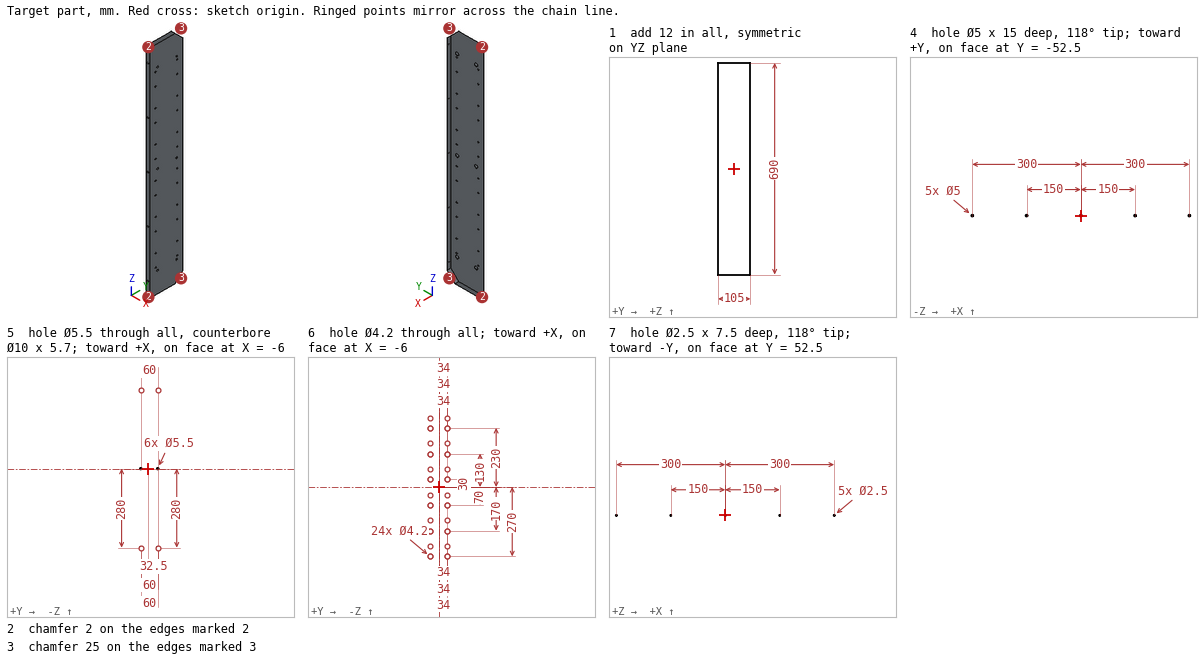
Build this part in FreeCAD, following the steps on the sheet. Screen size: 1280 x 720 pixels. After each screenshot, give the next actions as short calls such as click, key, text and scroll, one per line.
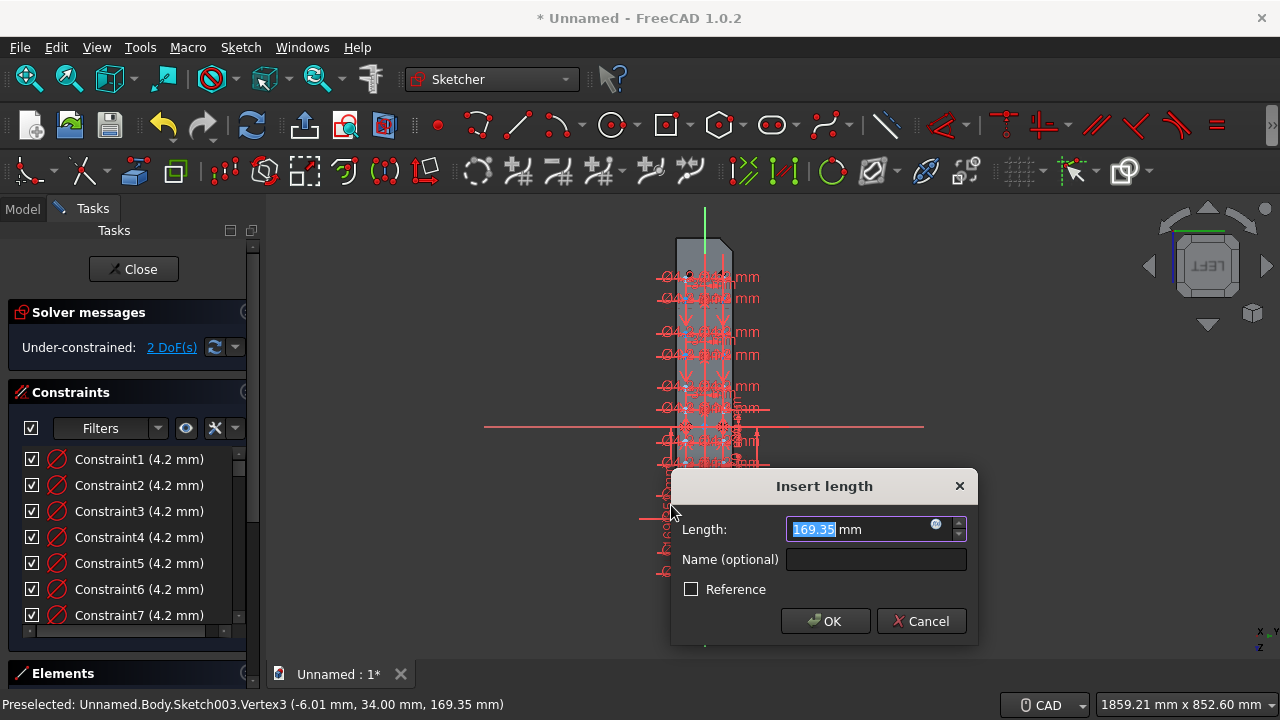
text(170)
key(Return)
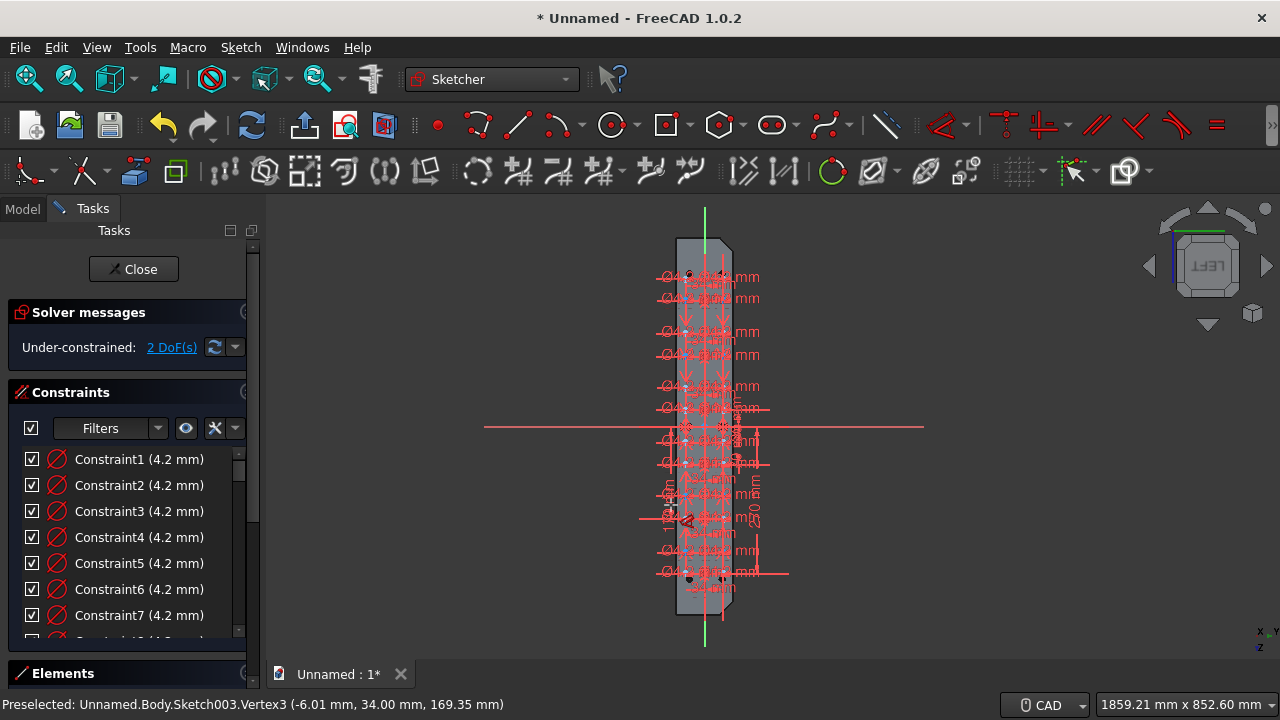
click(723, 357)
click(757, 367)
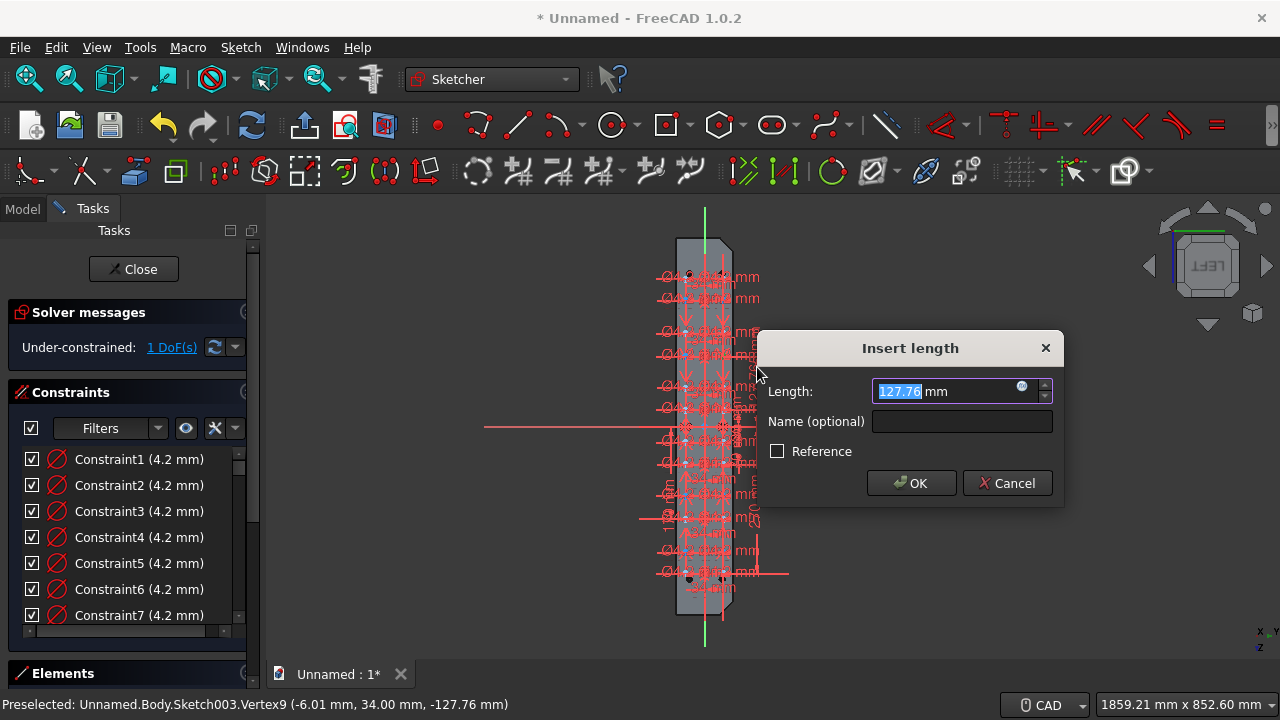
text(130)
key(Return)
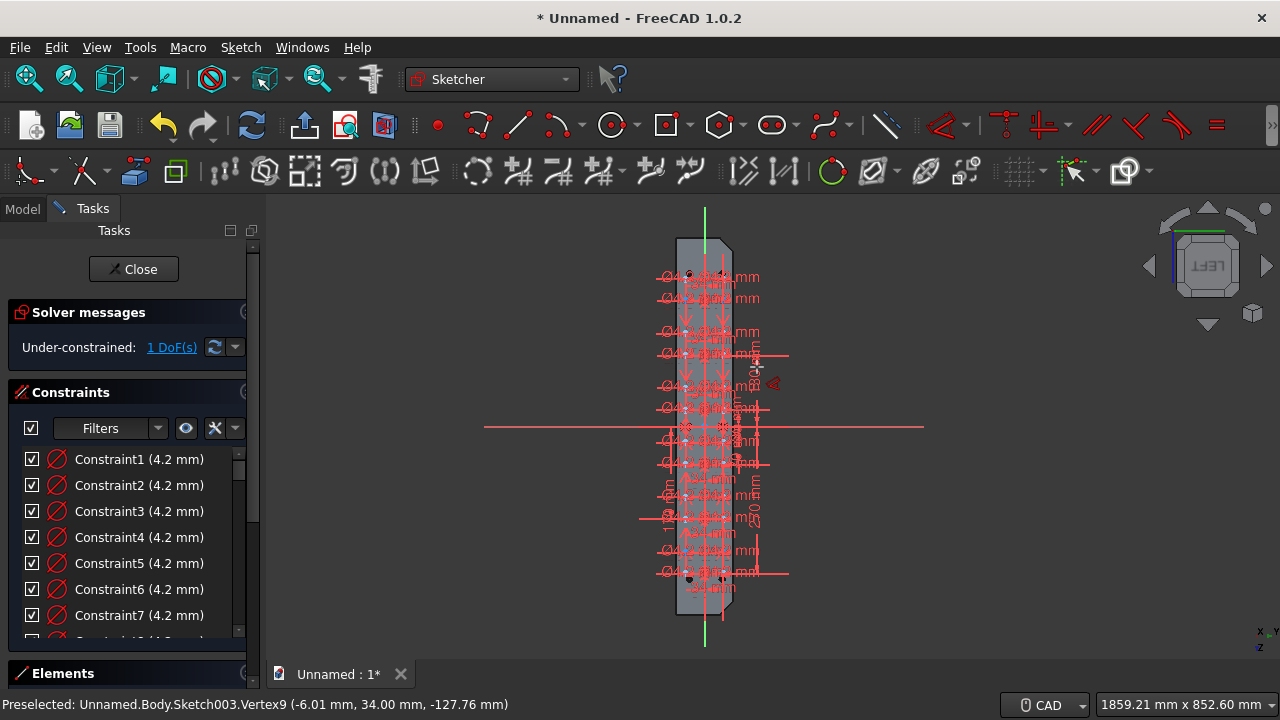
click(723, 301)
click(757, 319)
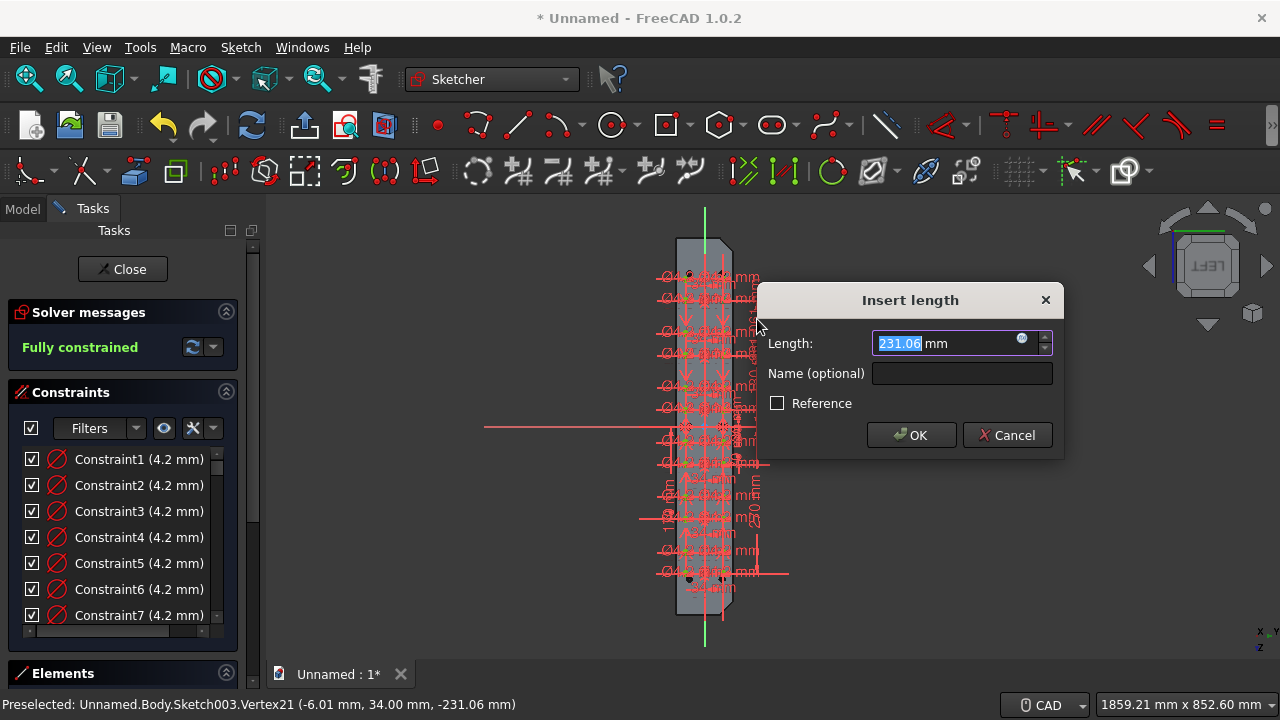
text(230)
key(Return)
key(Escape)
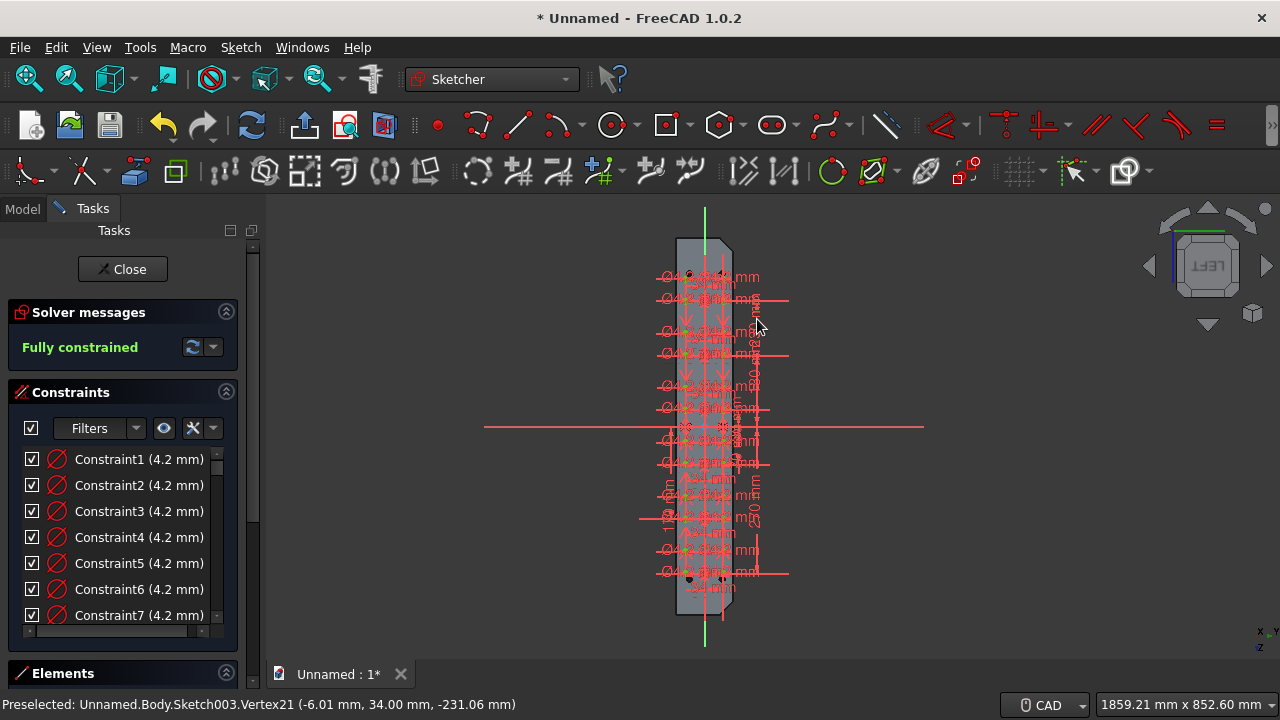
click(123, 269)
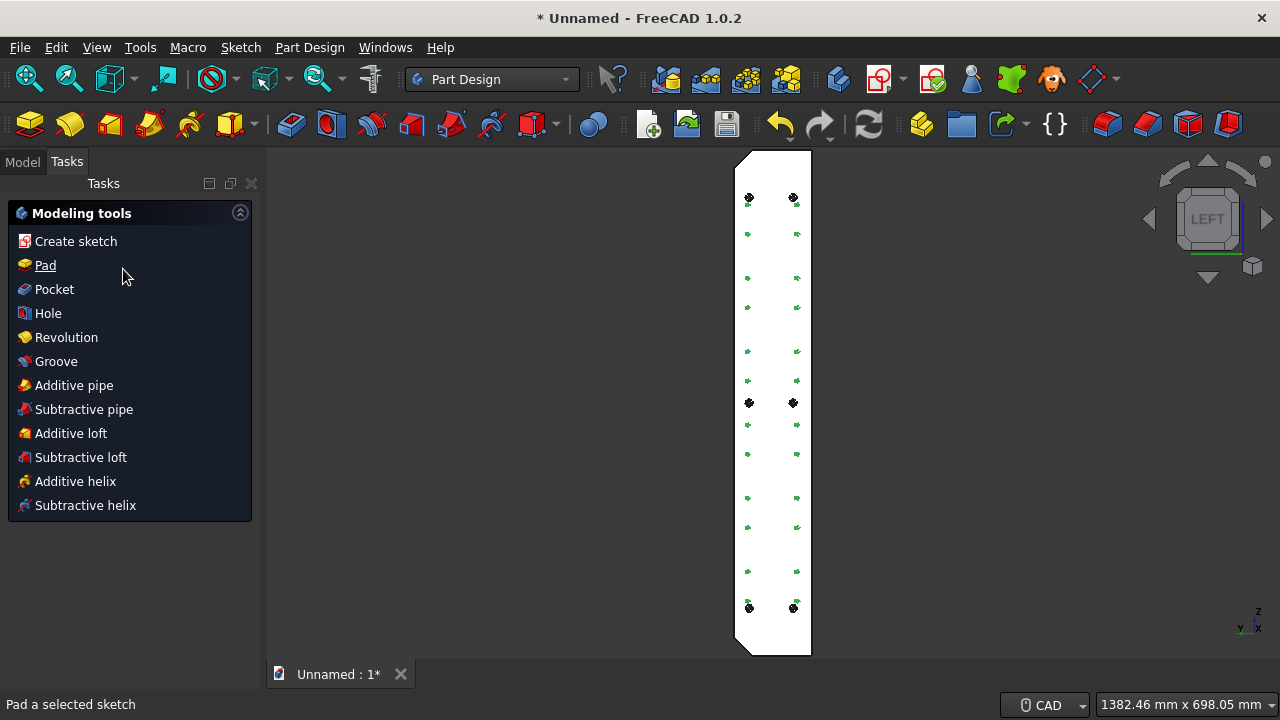
click(332, 124)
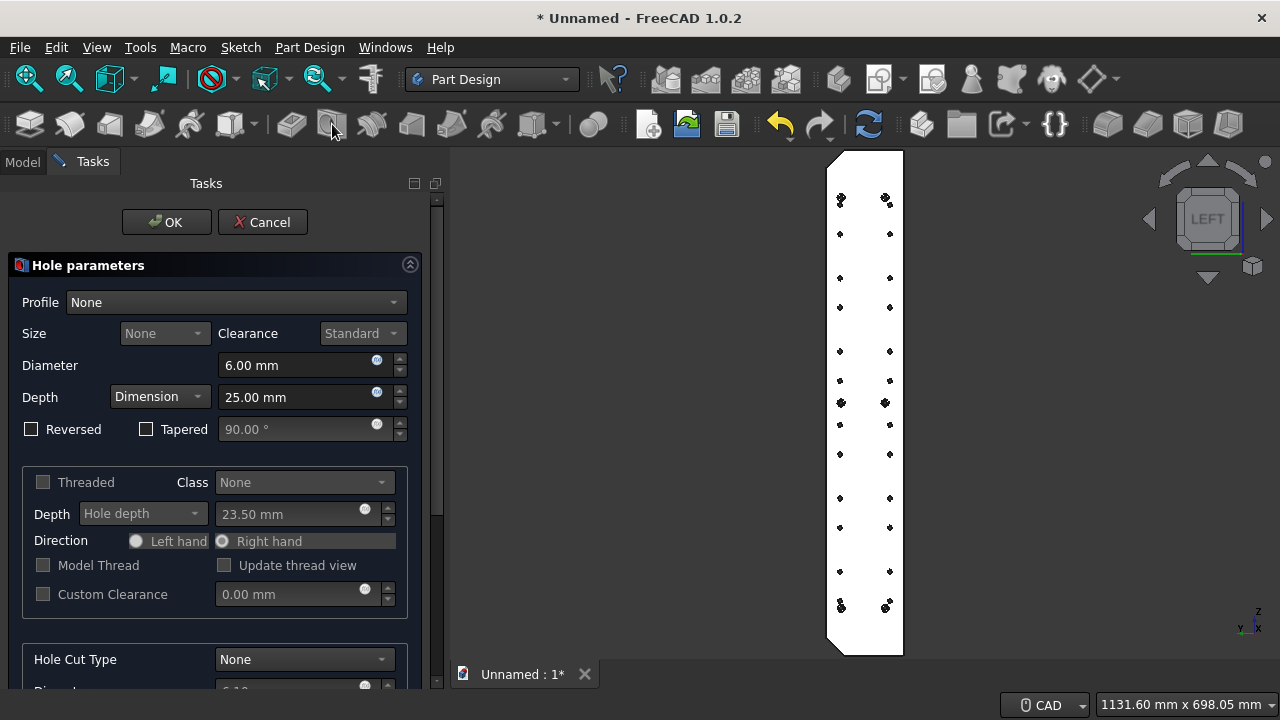
triple_click(305, 365)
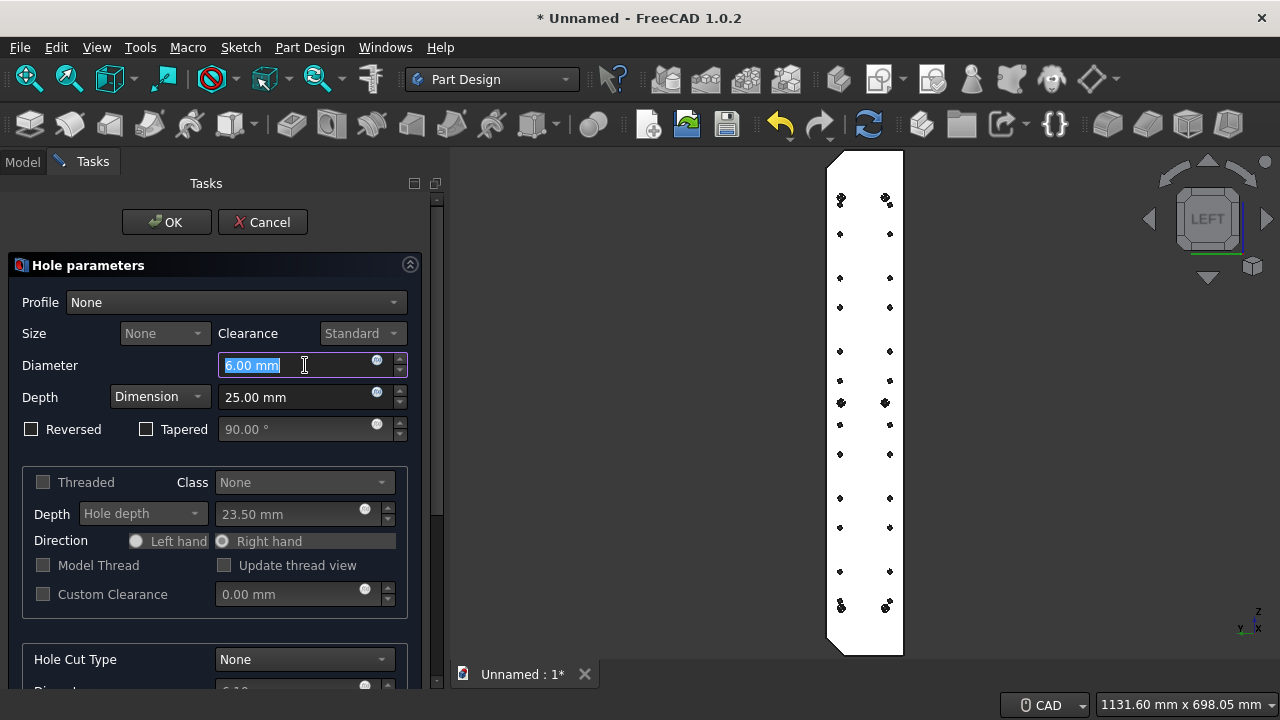
text(4.2)
key(Tab)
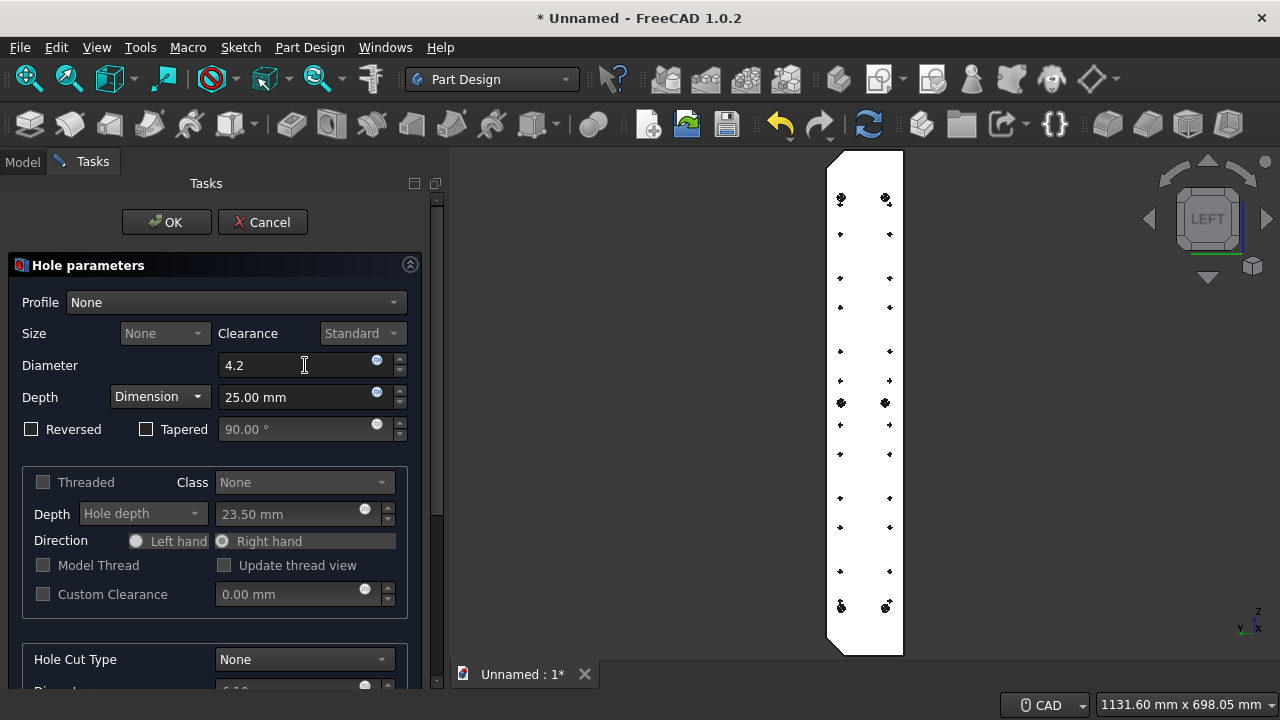
click(161, 396)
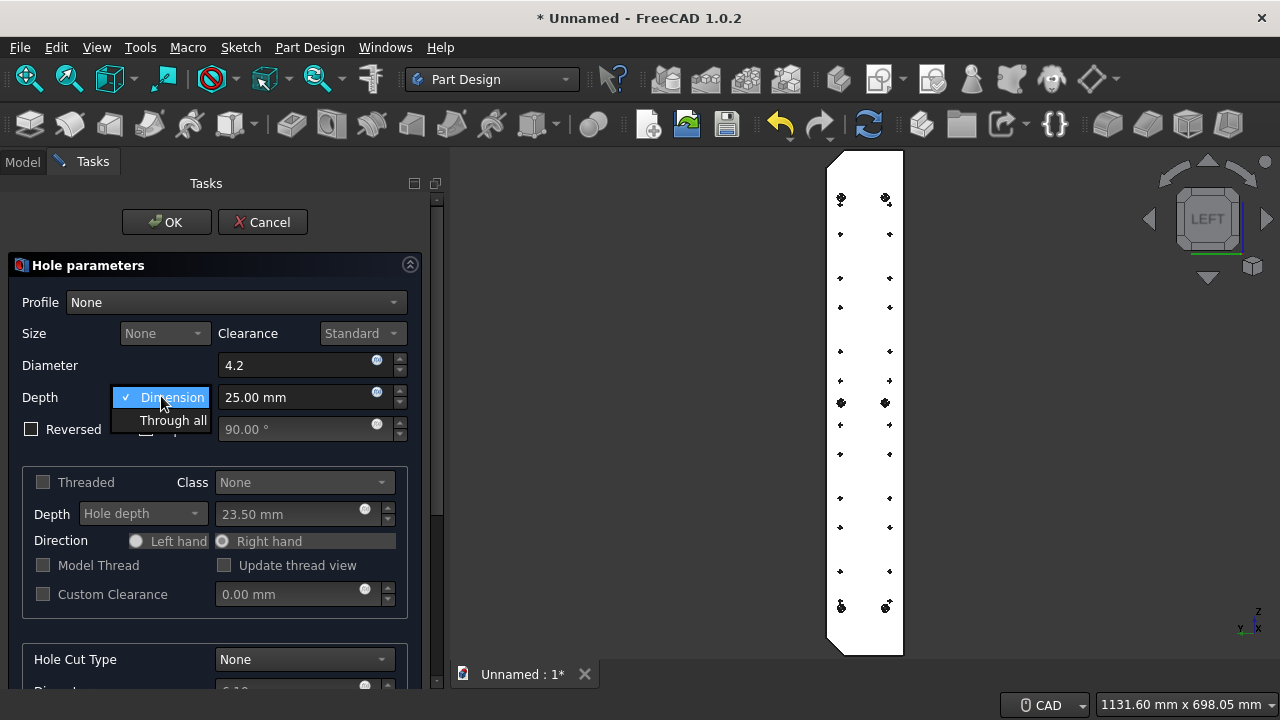
click(160, 420)